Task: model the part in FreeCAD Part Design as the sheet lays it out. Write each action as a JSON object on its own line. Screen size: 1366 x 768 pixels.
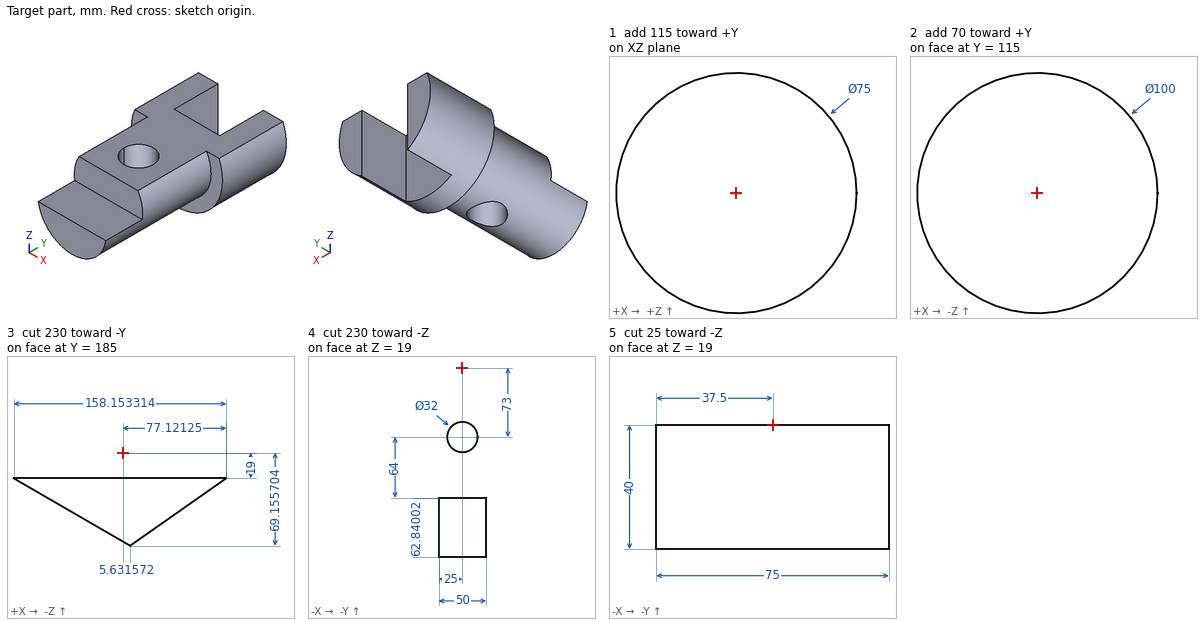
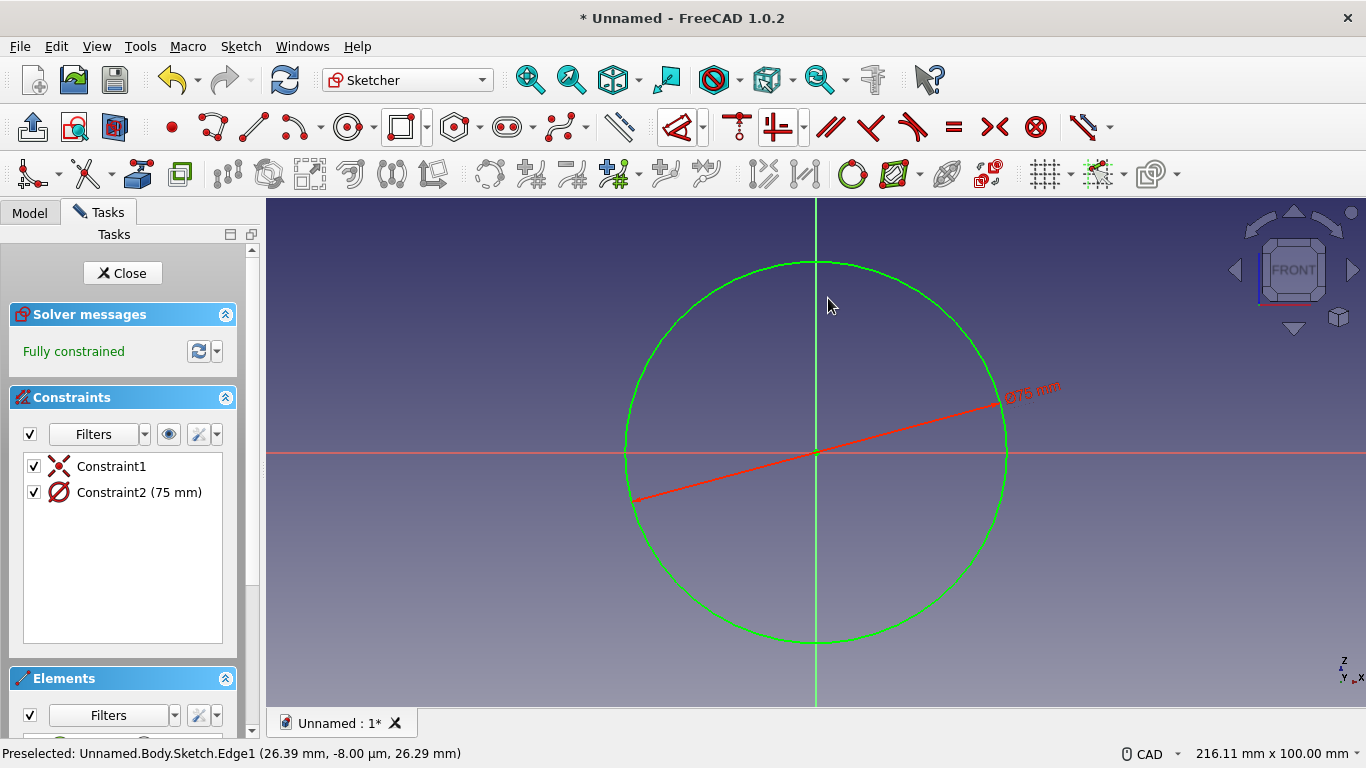
{"action": "left_click", "coordinate": [123, 273]}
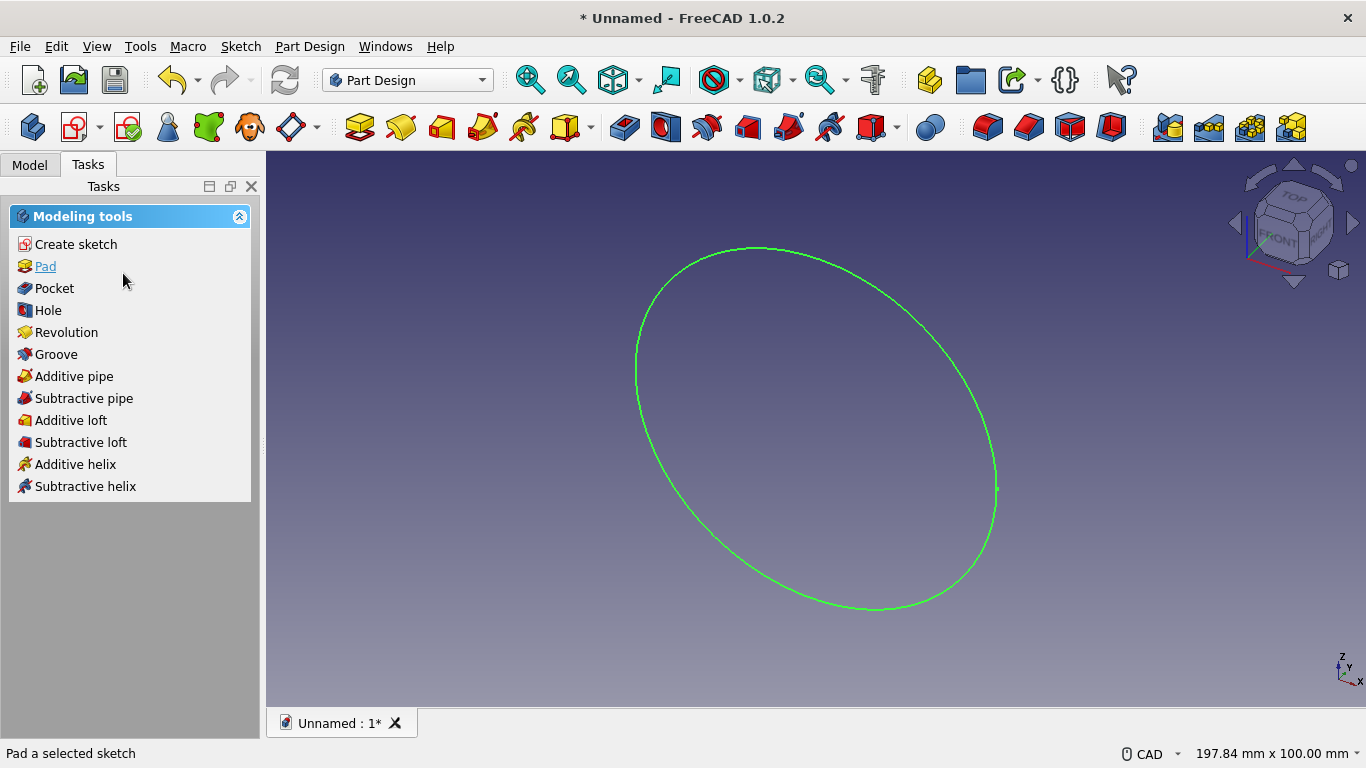
{"action": "left_click", "coordinate": [360, 128]}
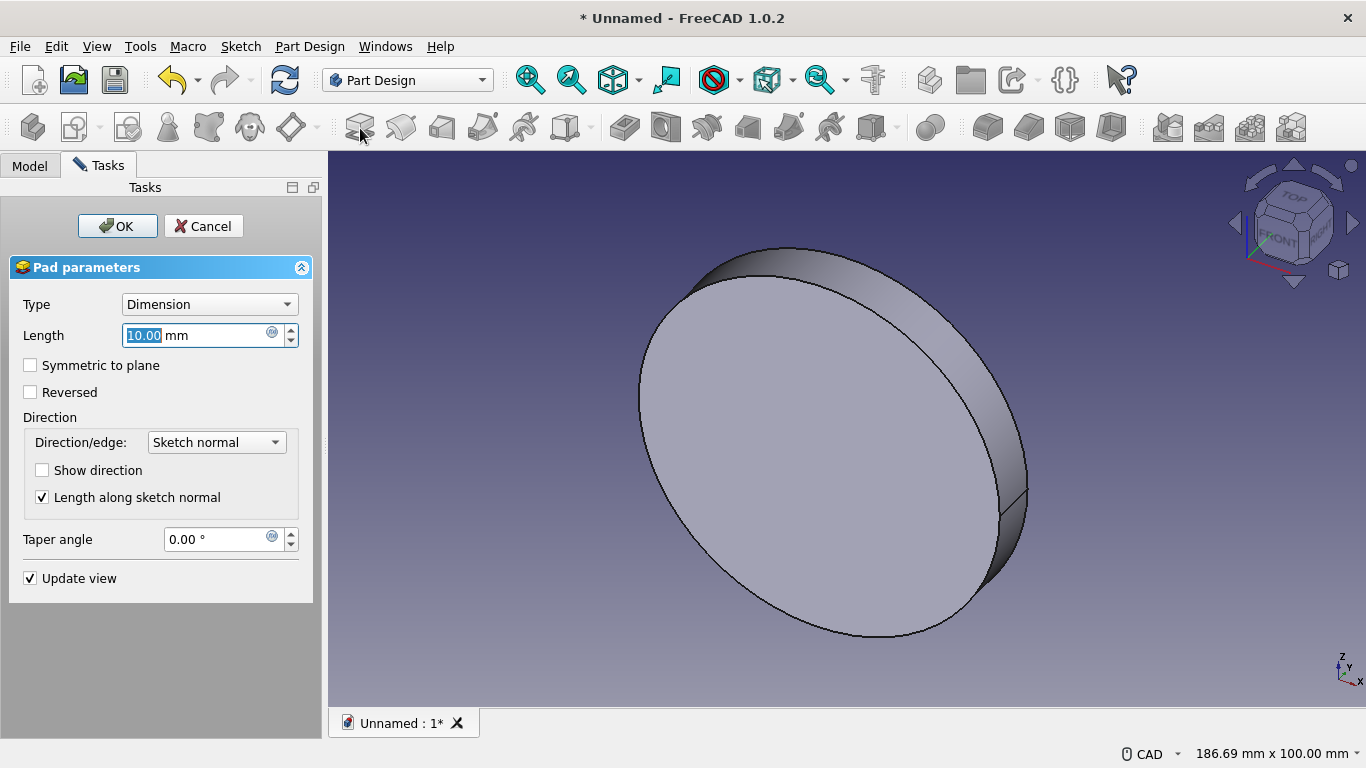
{"action": "type", "text": "115"}
{"action": "key", "text": "Tab"}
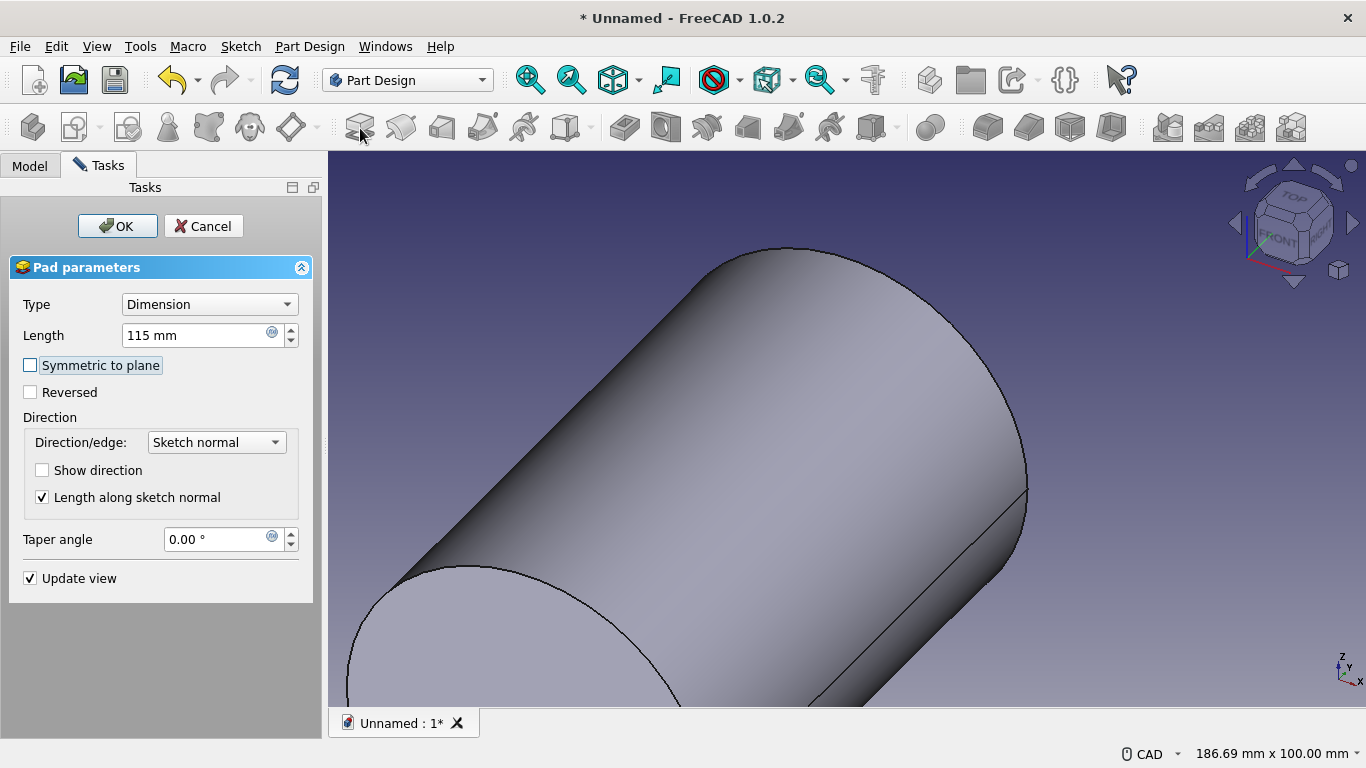
{"action": "left_click", "coordinate": [31, 392]}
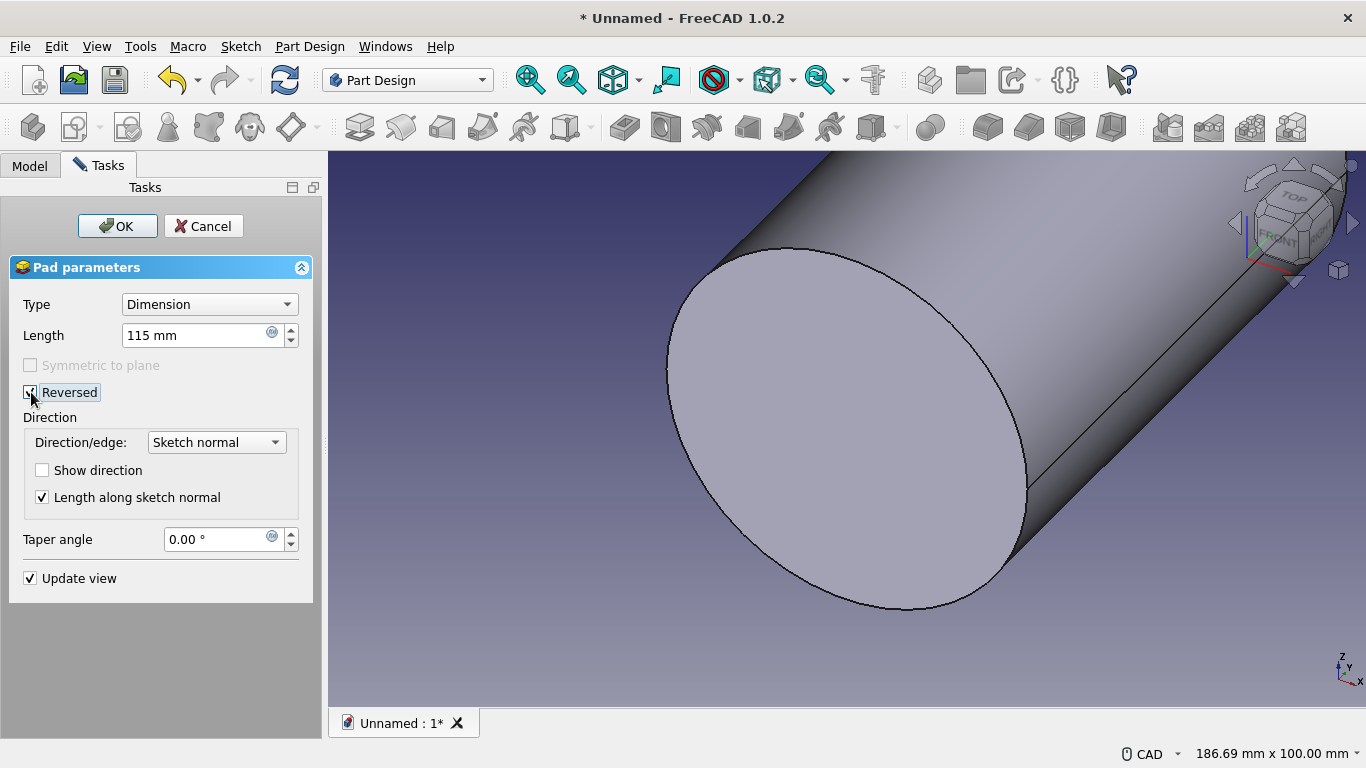
{"action": "left_click", "coordinate": [118, 226]}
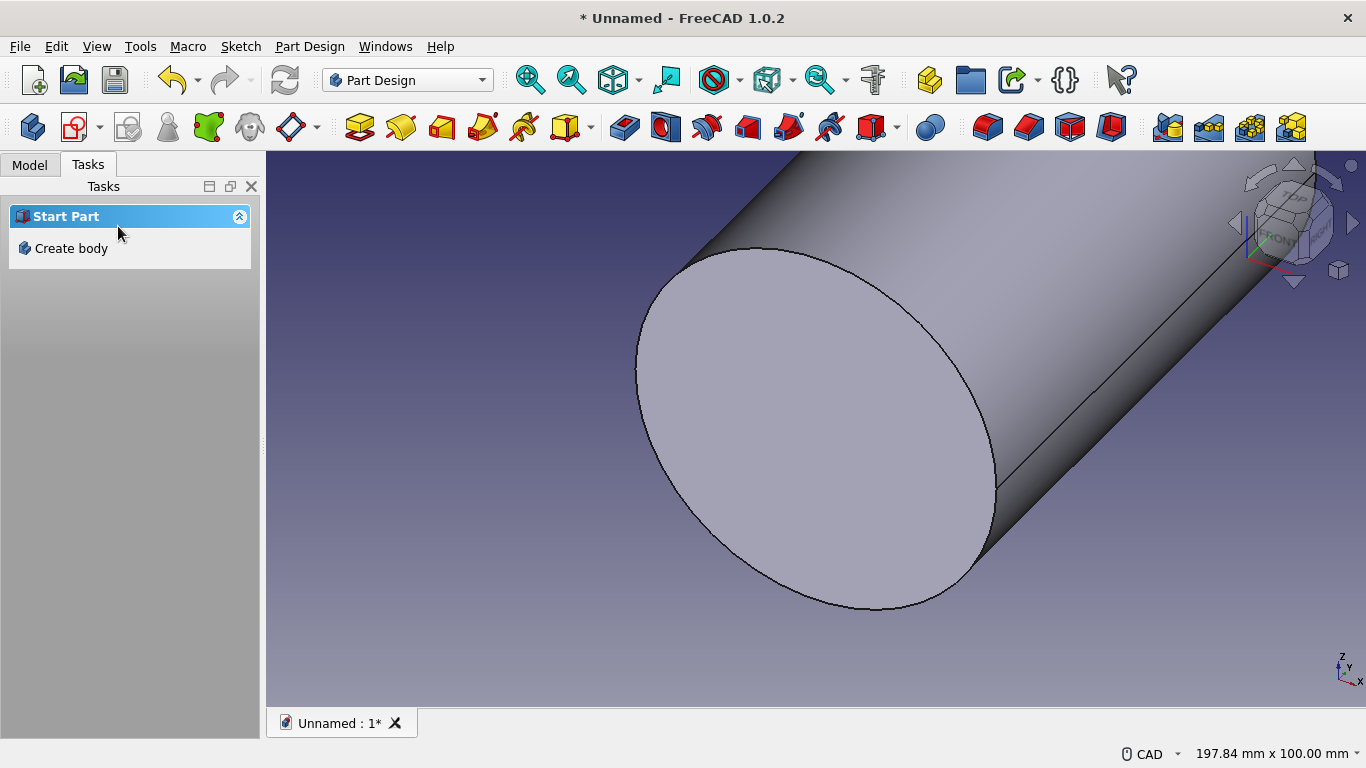
{"action": "left_click", "coordinate": [531, 80]}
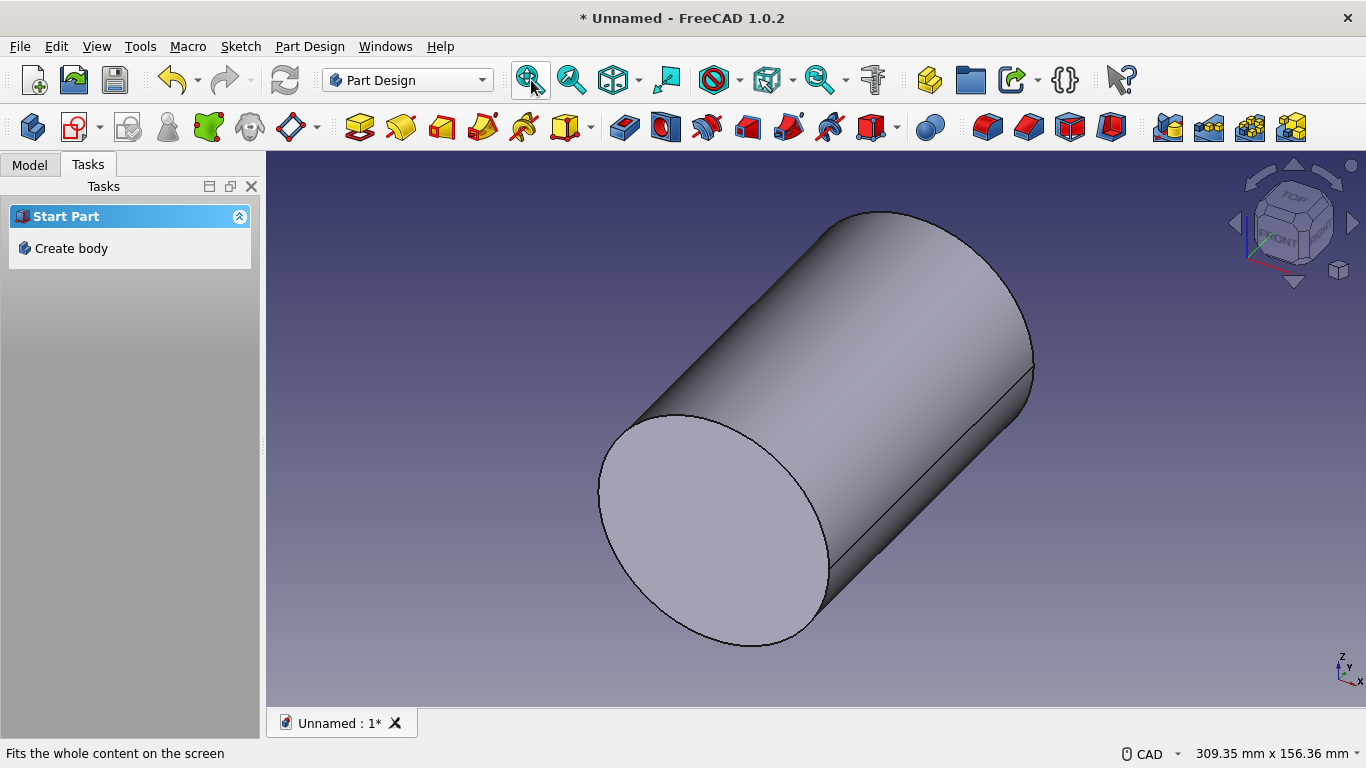
{"action": "key", "text": "4"}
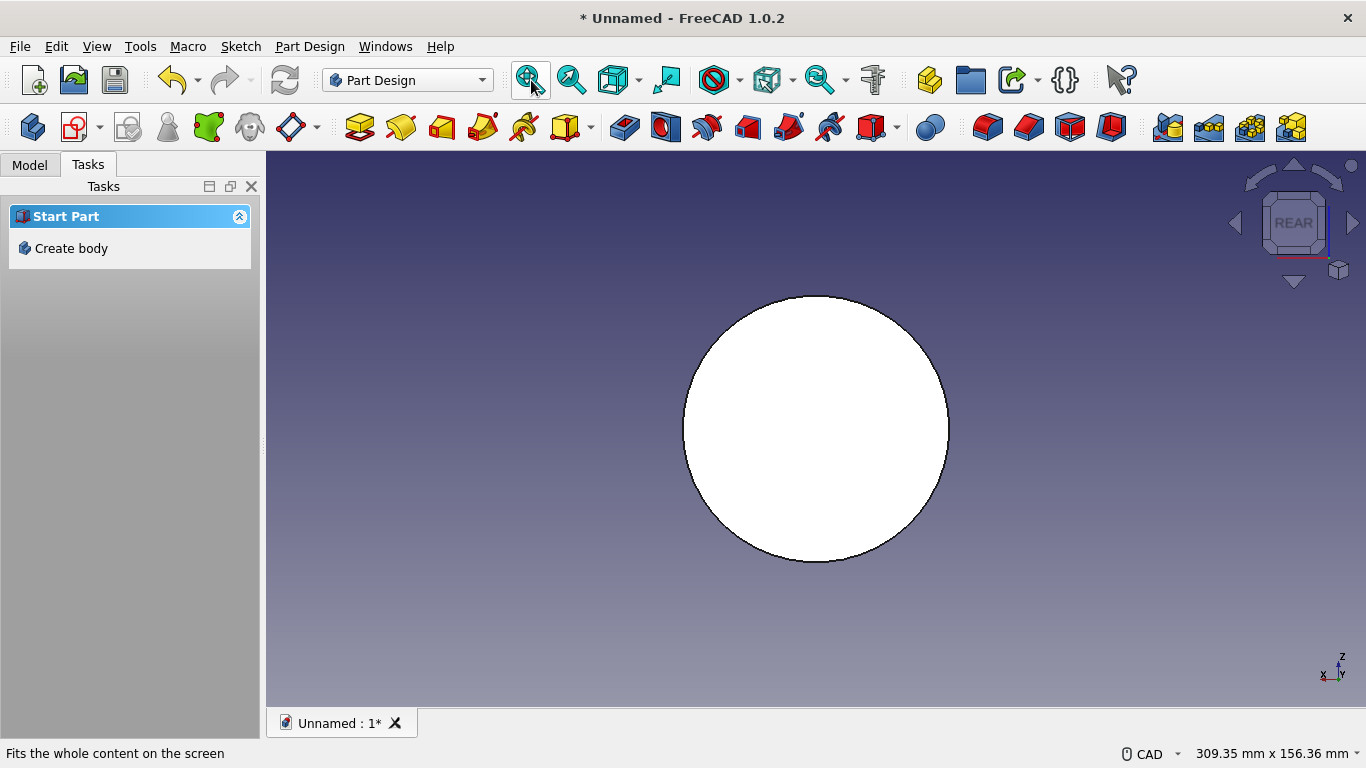
{"action": "left_click", "coordinate": [816, 428]}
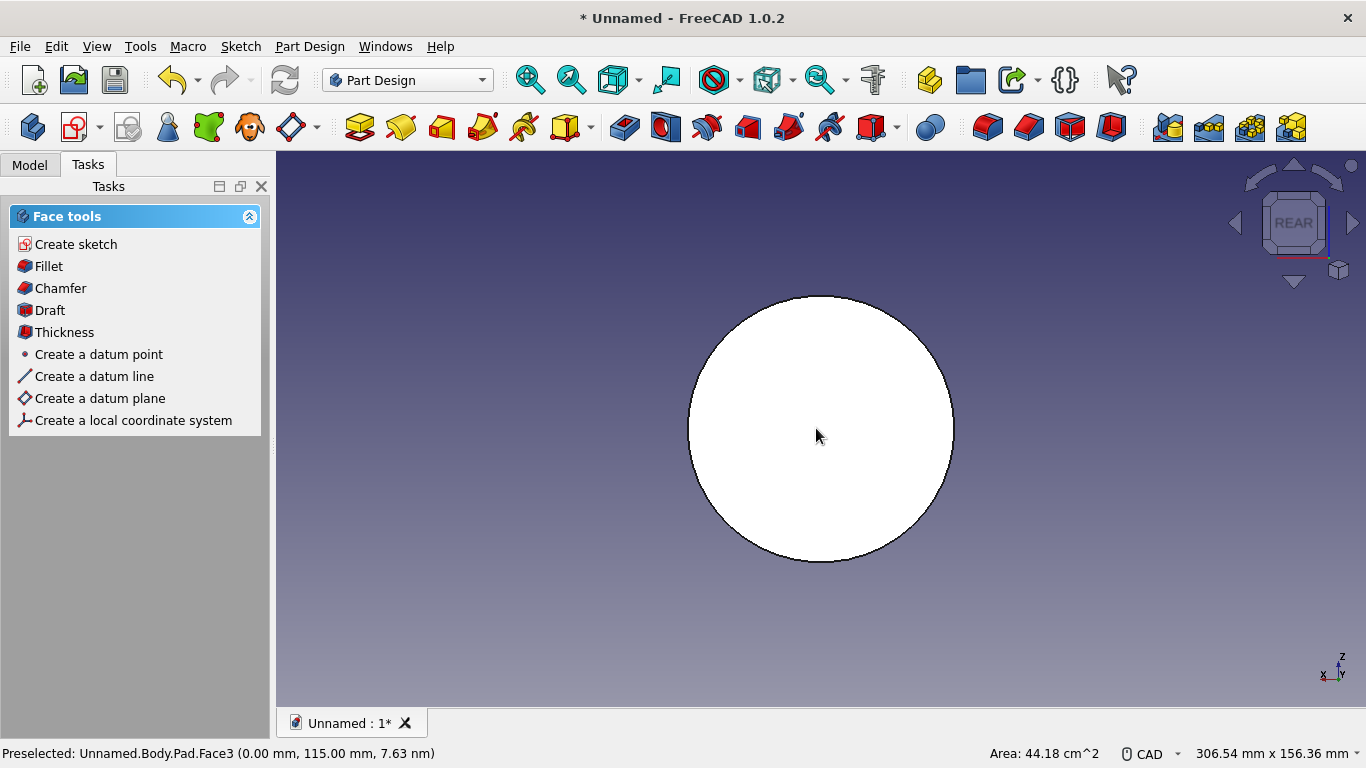
{"action": "left_click", "coordinate": [74, 128]}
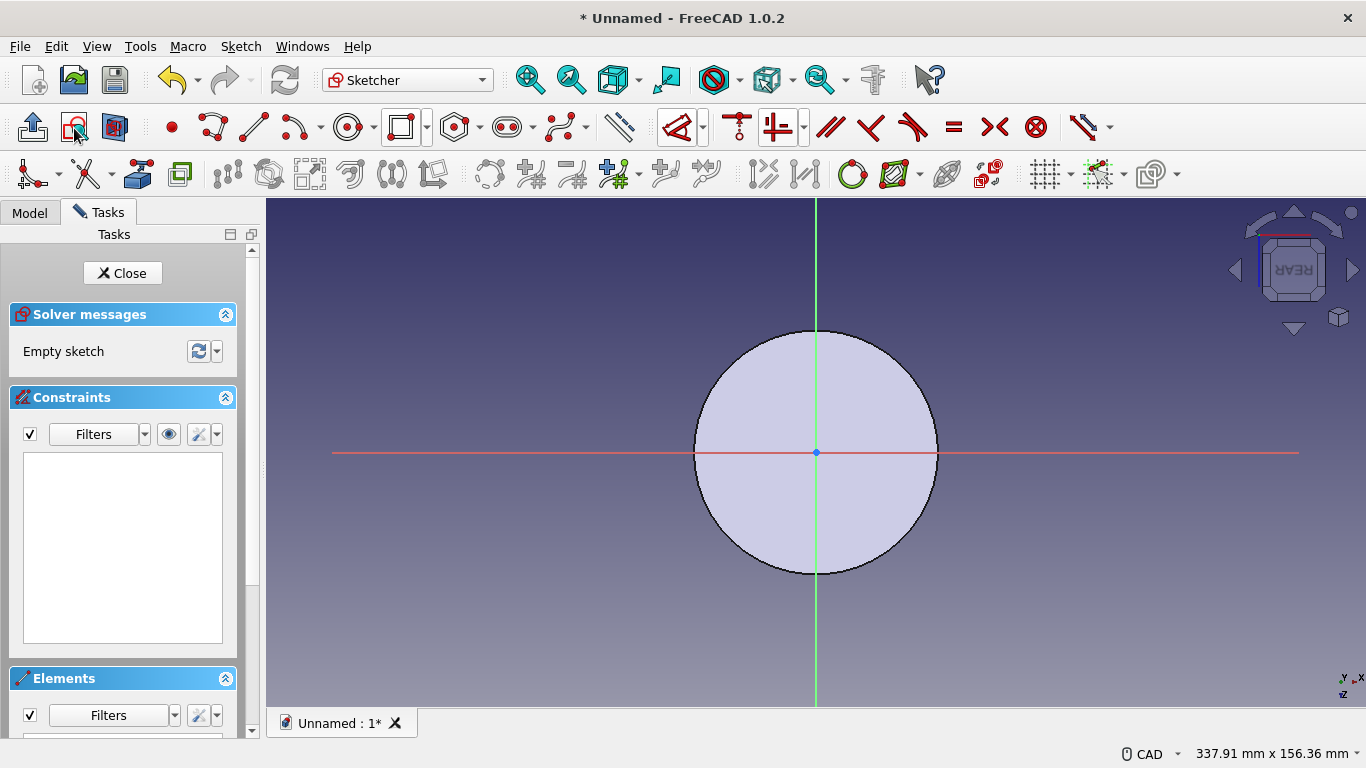
{"action": "left_click", "coordinate": [348, 128]}